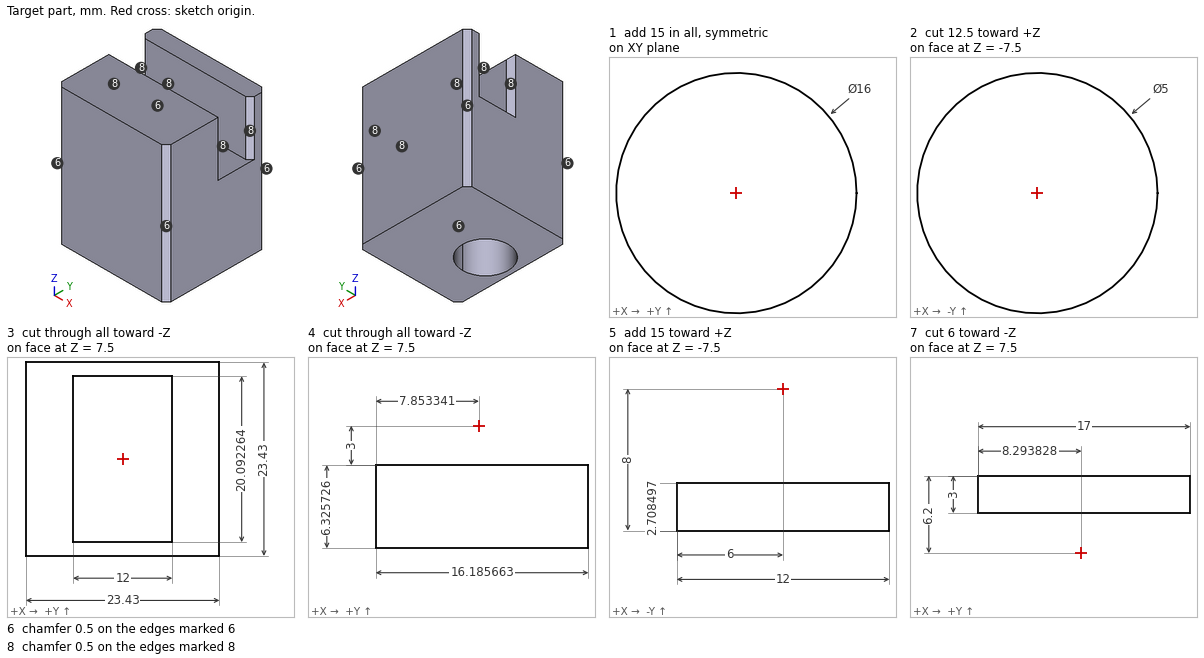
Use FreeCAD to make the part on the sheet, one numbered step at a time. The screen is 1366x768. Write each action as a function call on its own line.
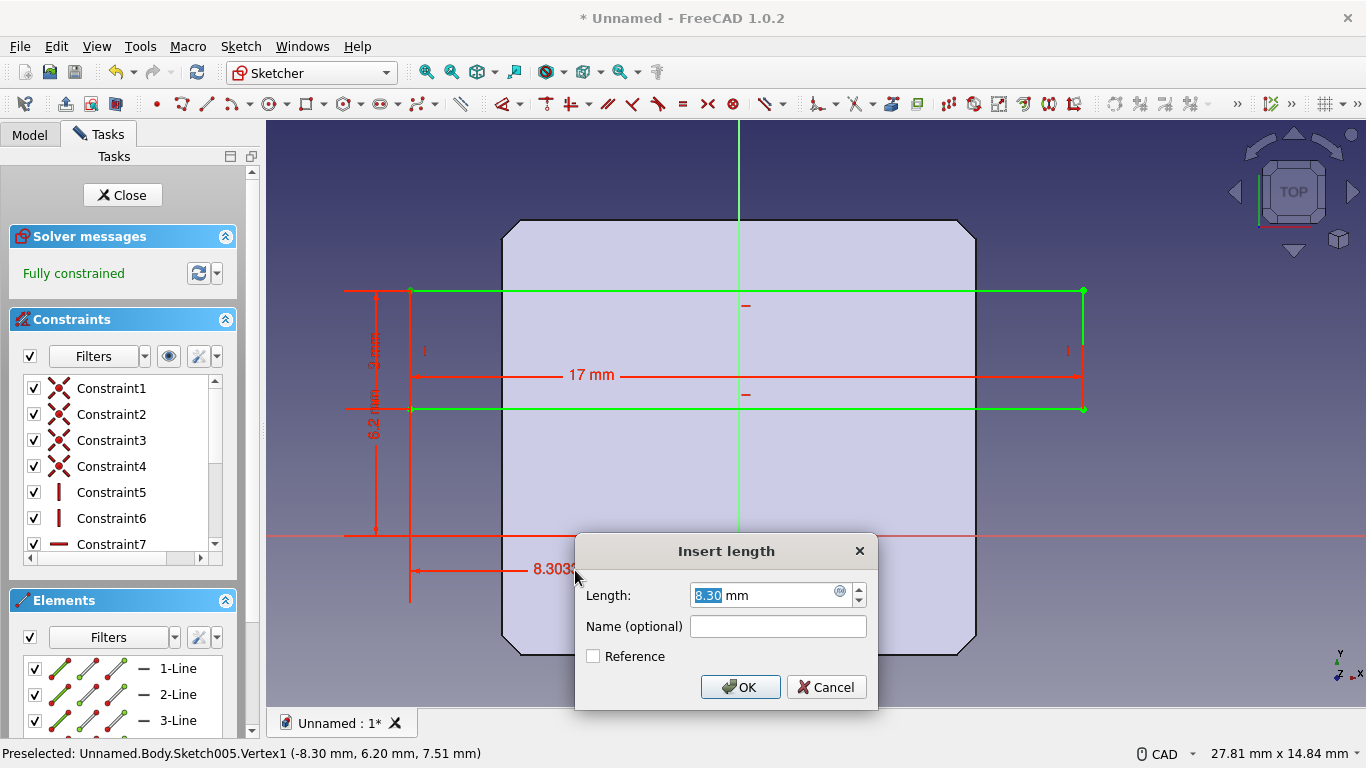
text(8.293828)
key(Return)
key(Escape)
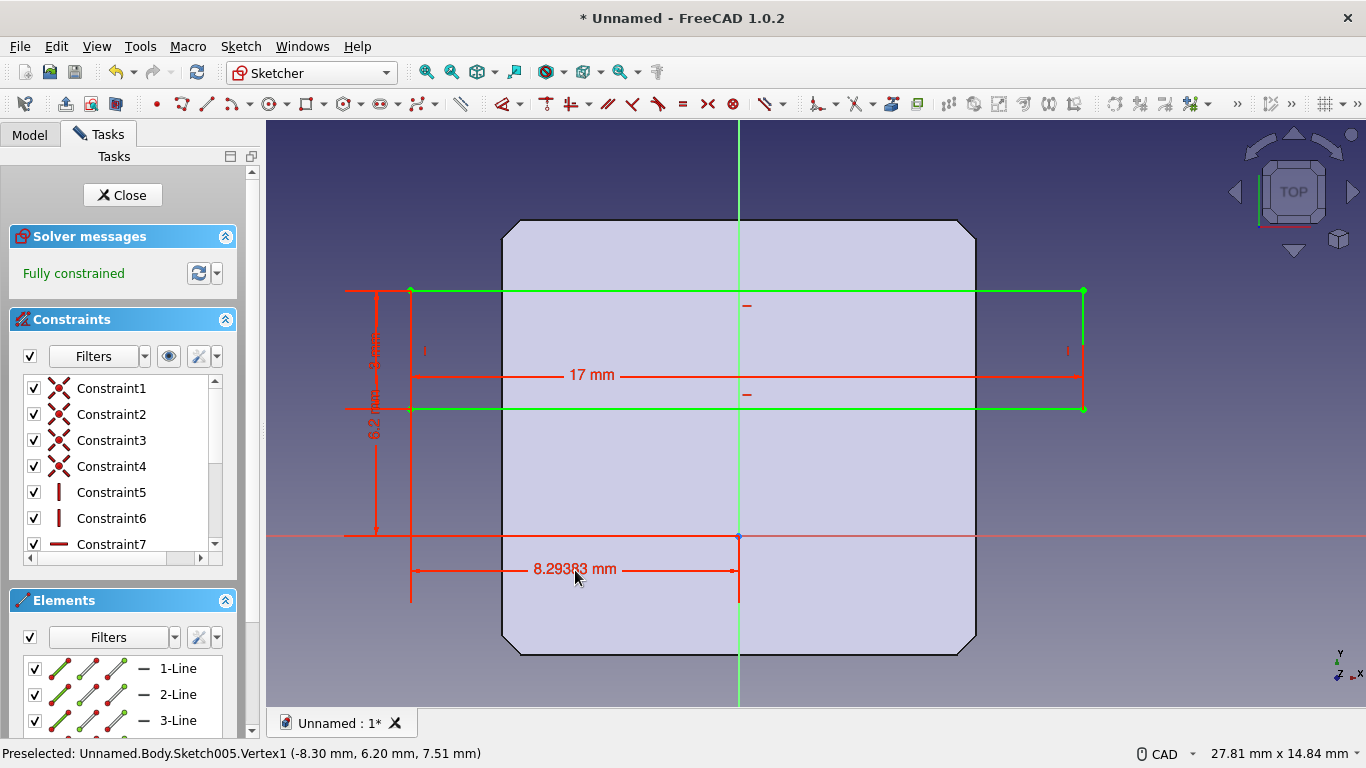
click(123, 195)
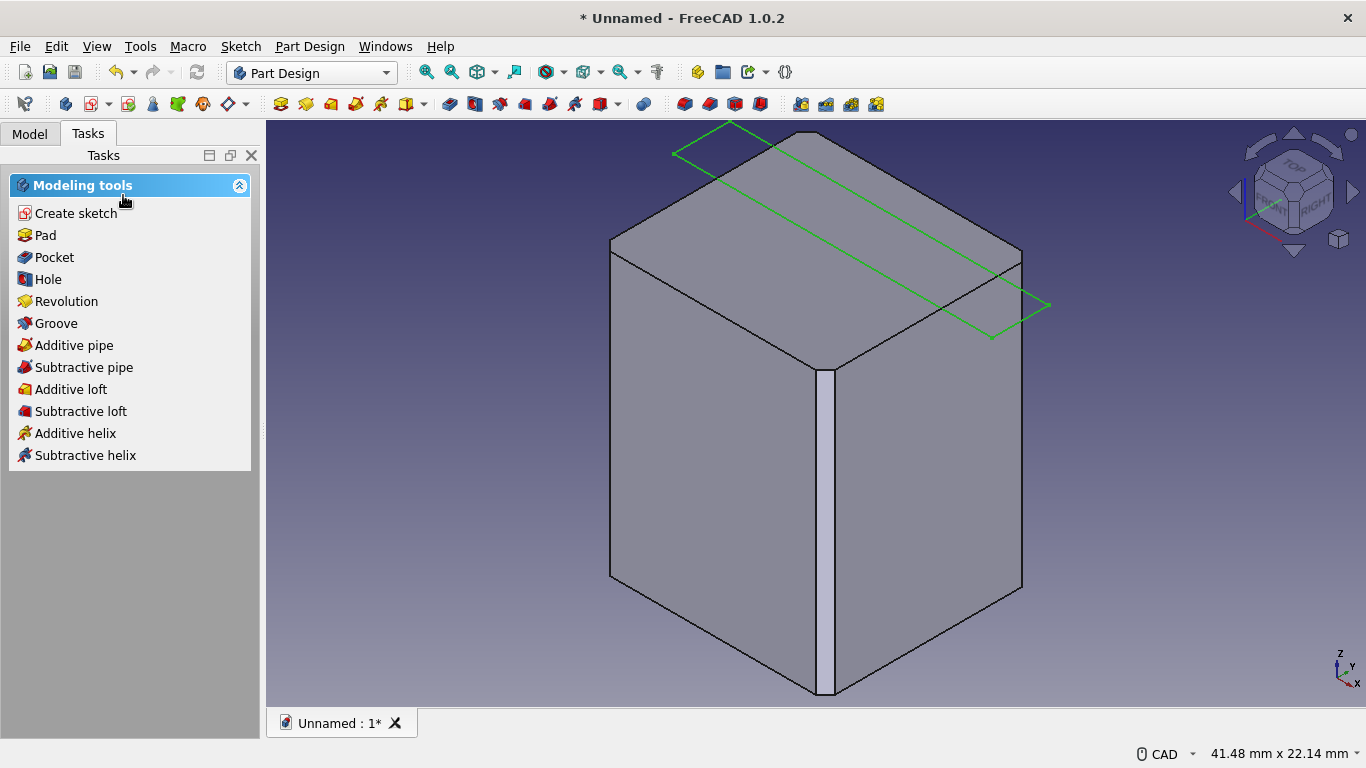
click(450, 104)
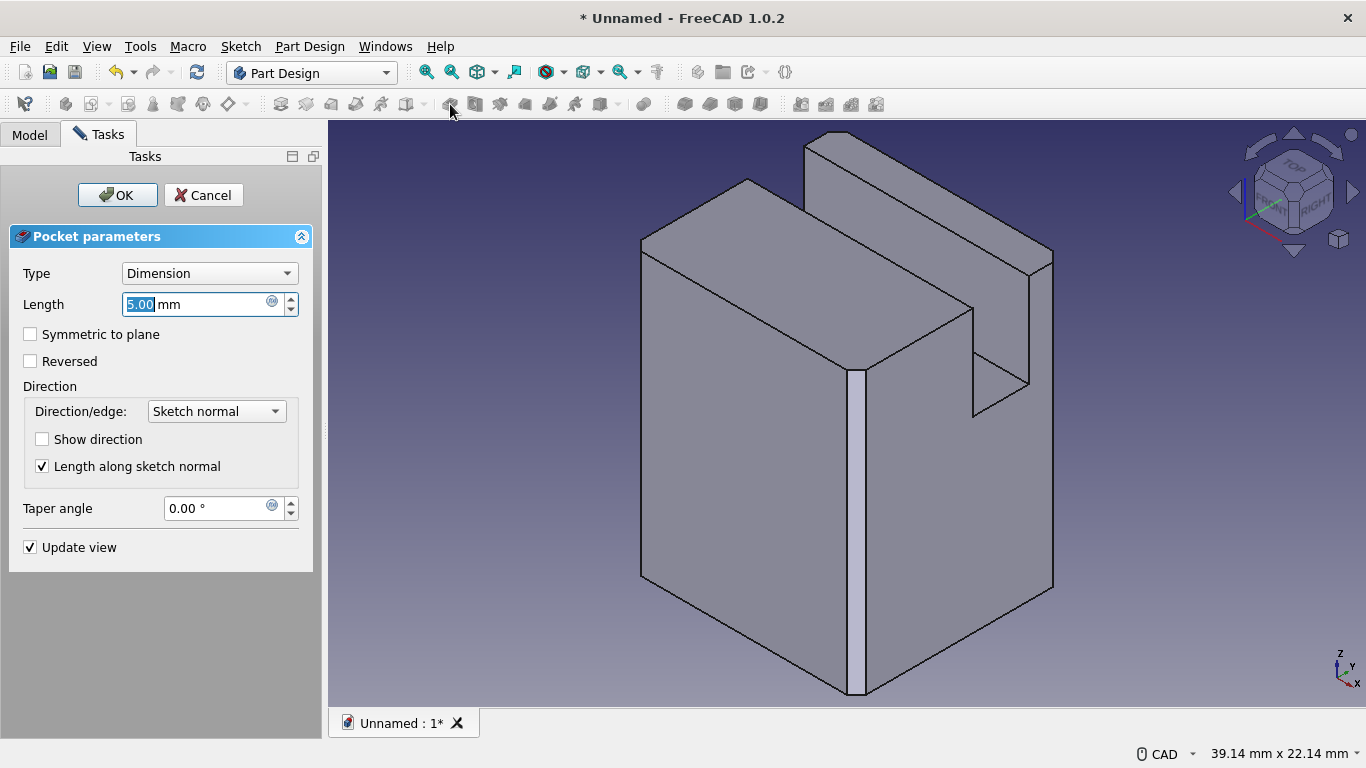
text(6)
key(Tab)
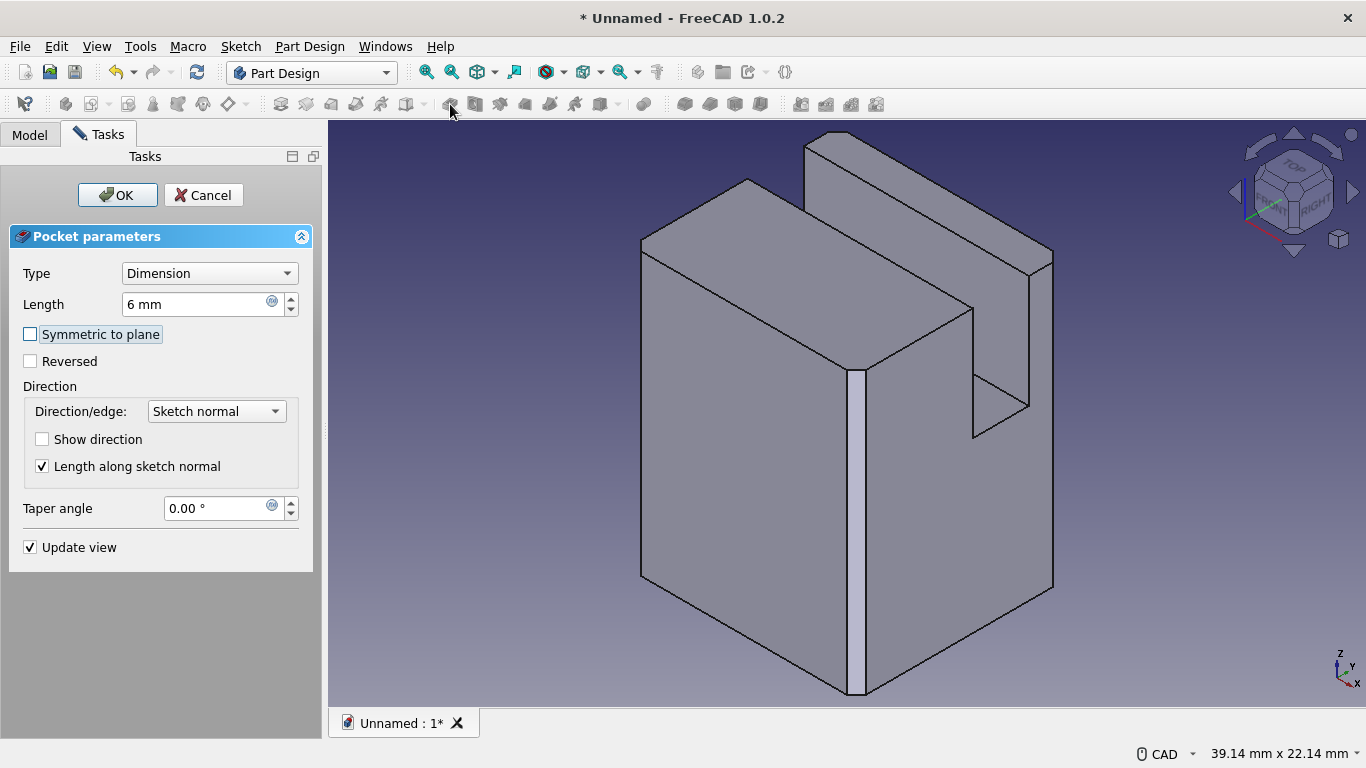
click(118, 195)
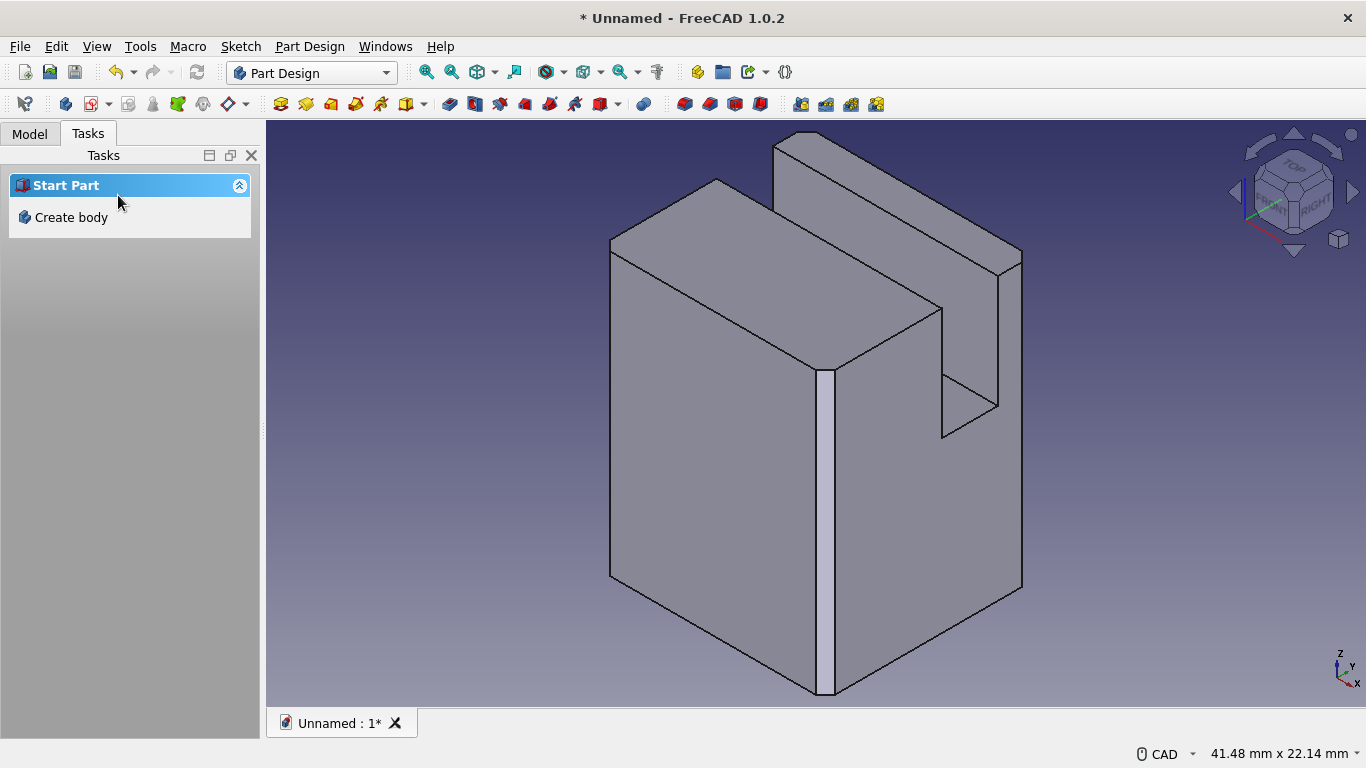
click(998, 340)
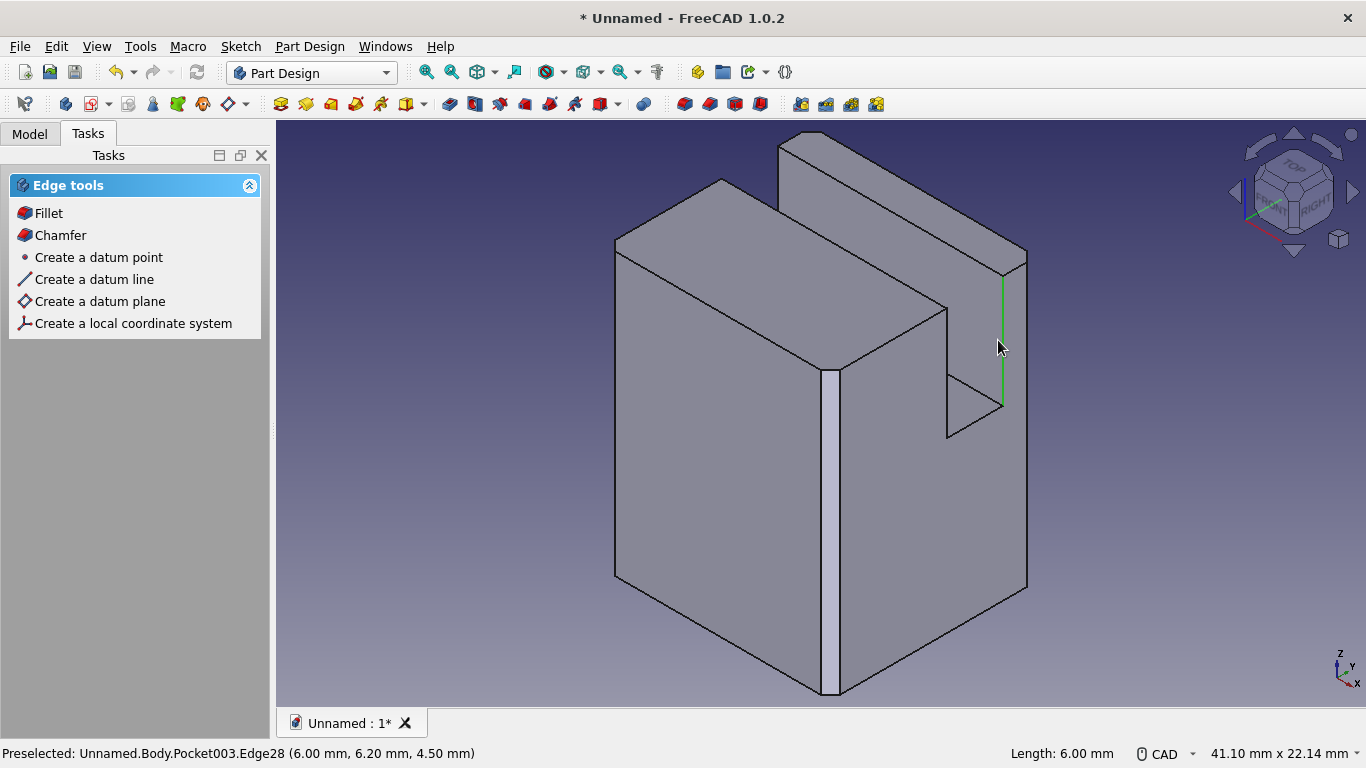
key(2)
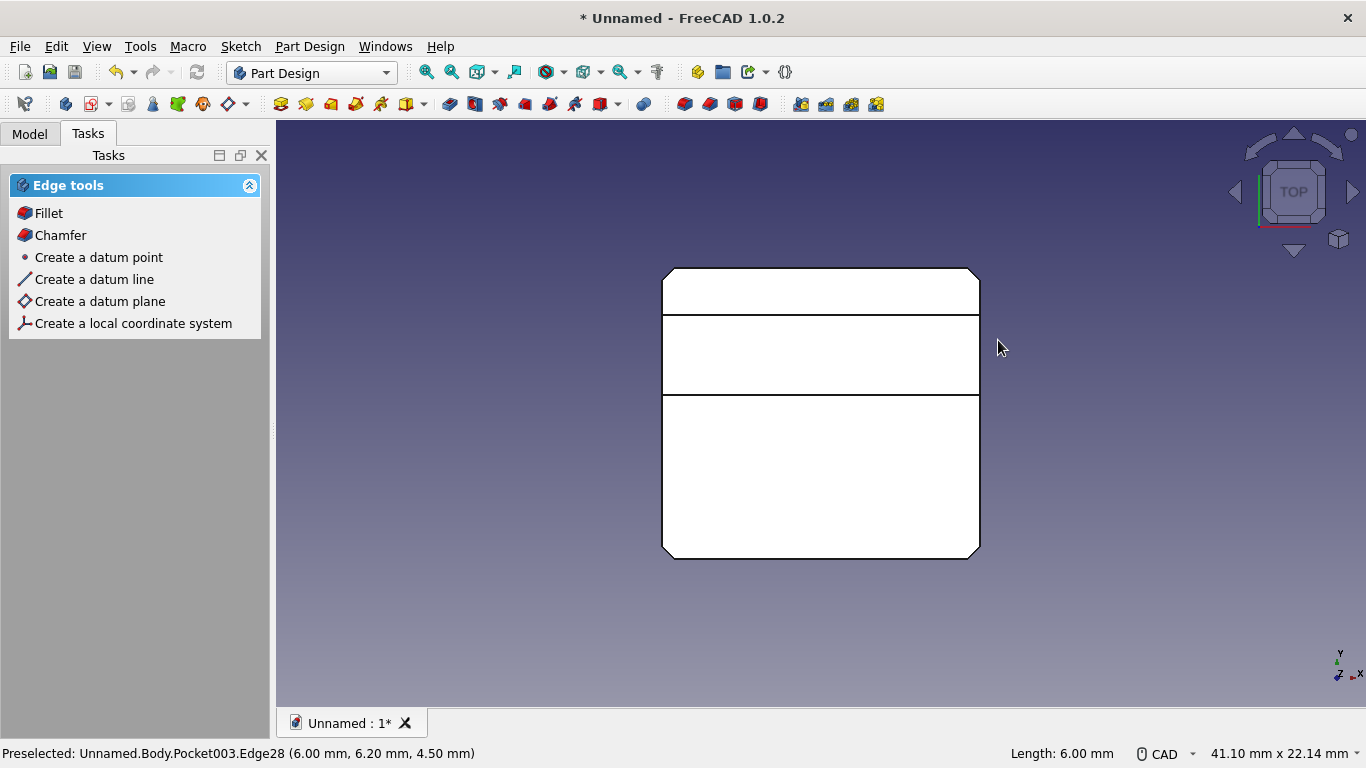
click(821, 394, ctrl)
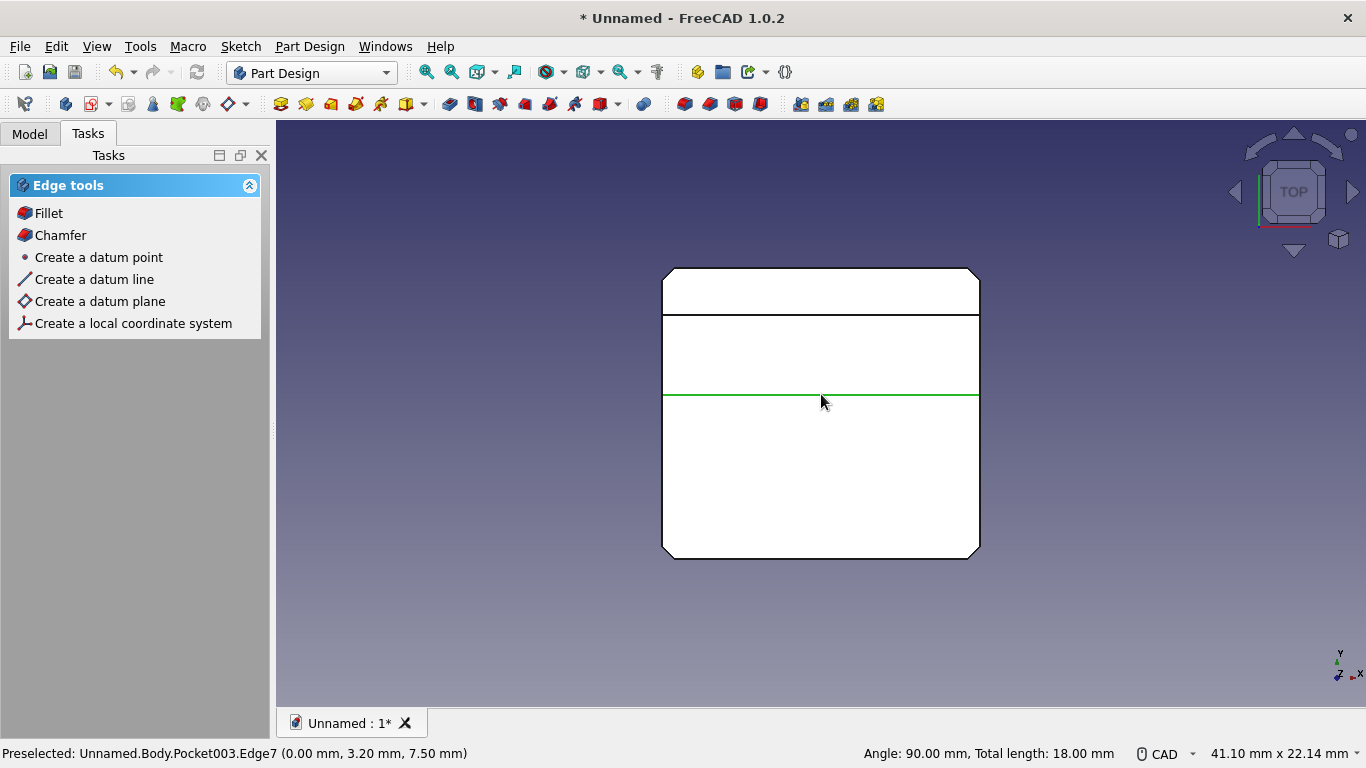
key(0)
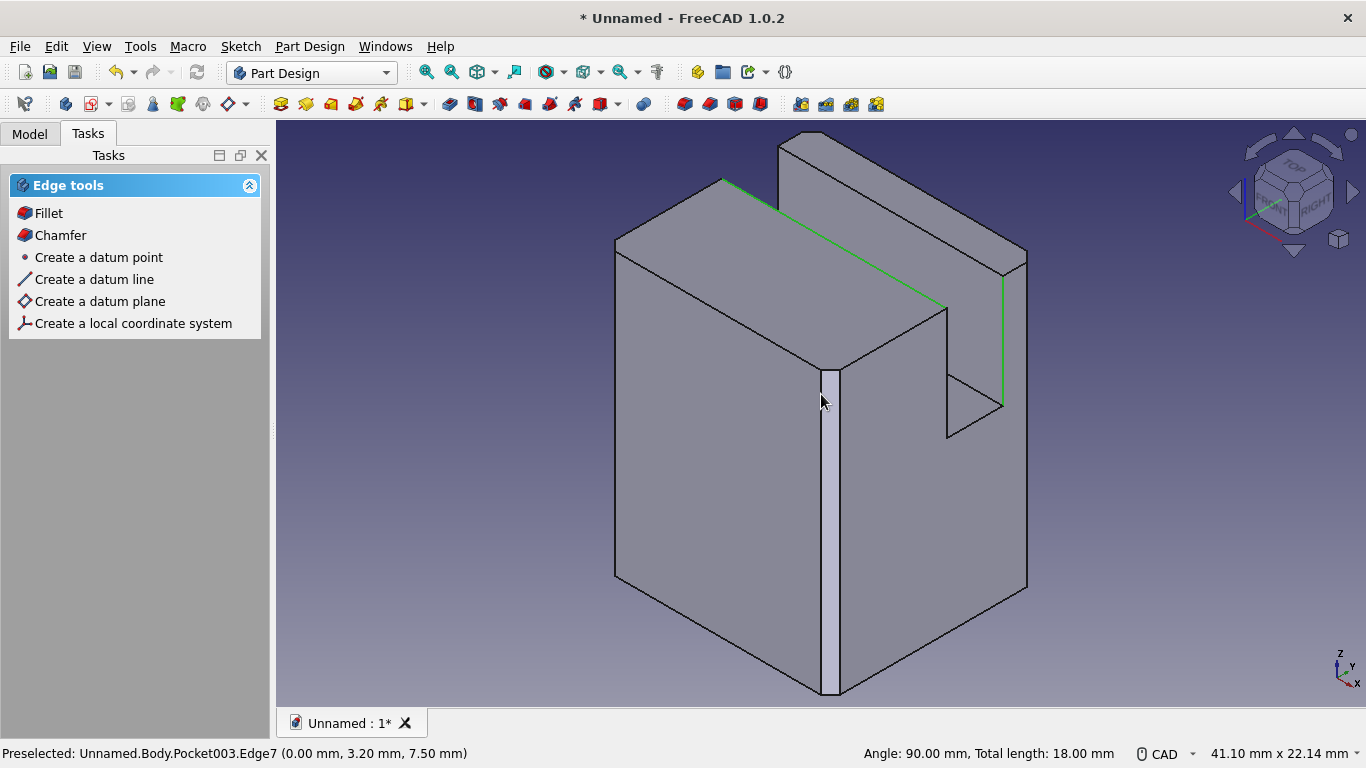
key(1)